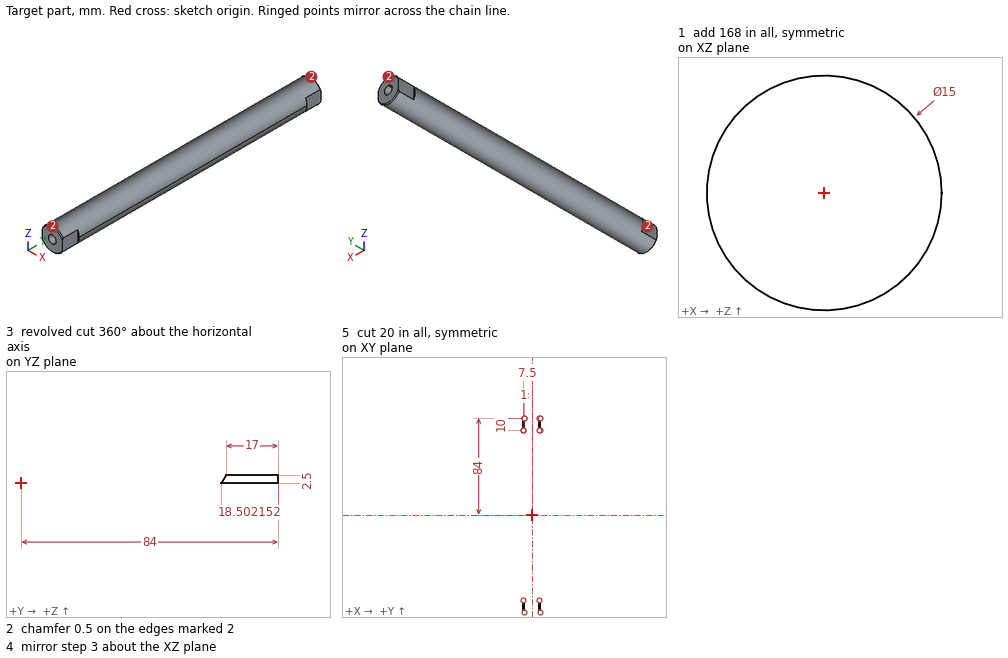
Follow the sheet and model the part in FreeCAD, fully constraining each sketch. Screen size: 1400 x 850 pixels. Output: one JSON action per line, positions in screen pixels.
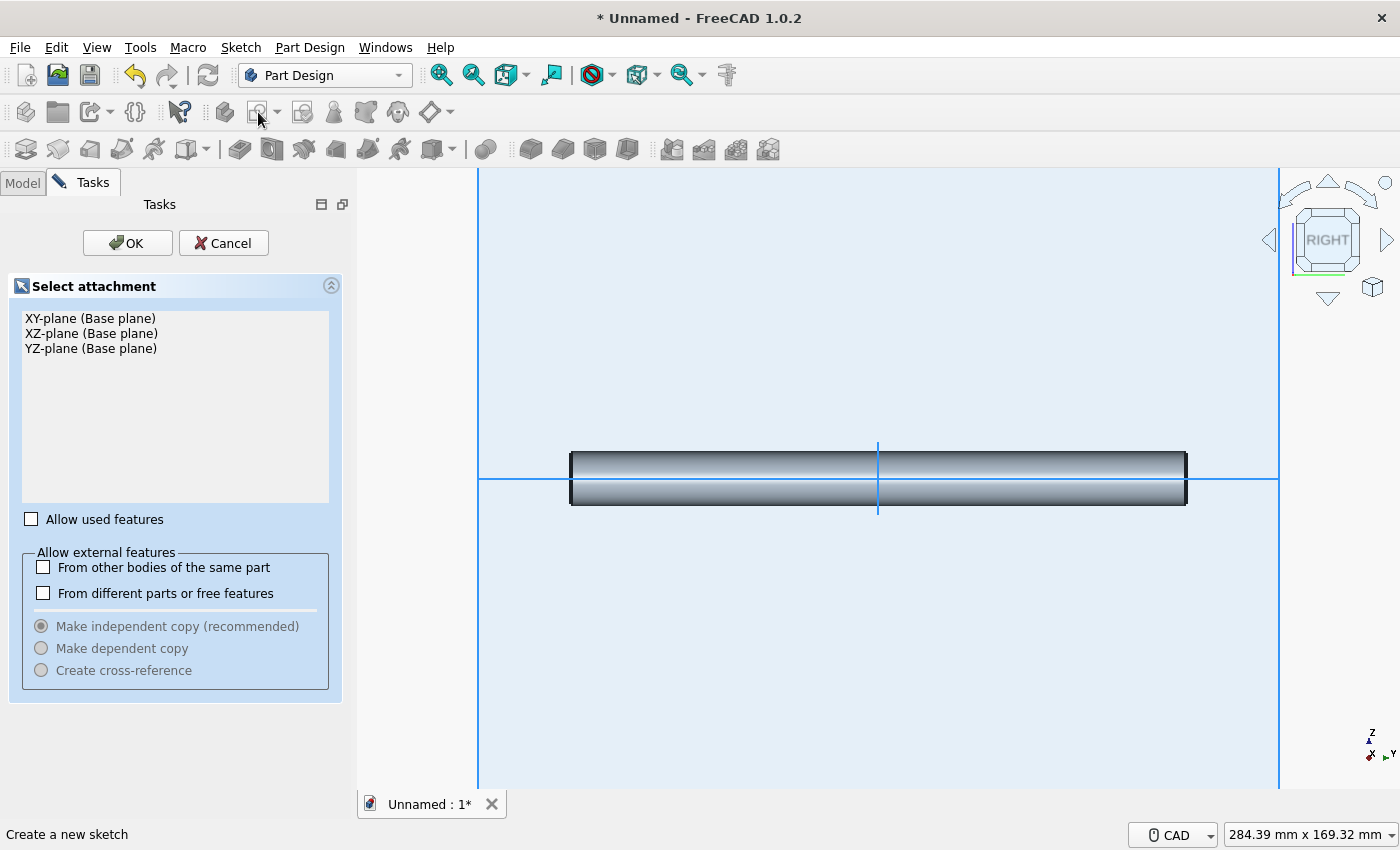
{"action": "left_click", "coordinate": [82, 348]}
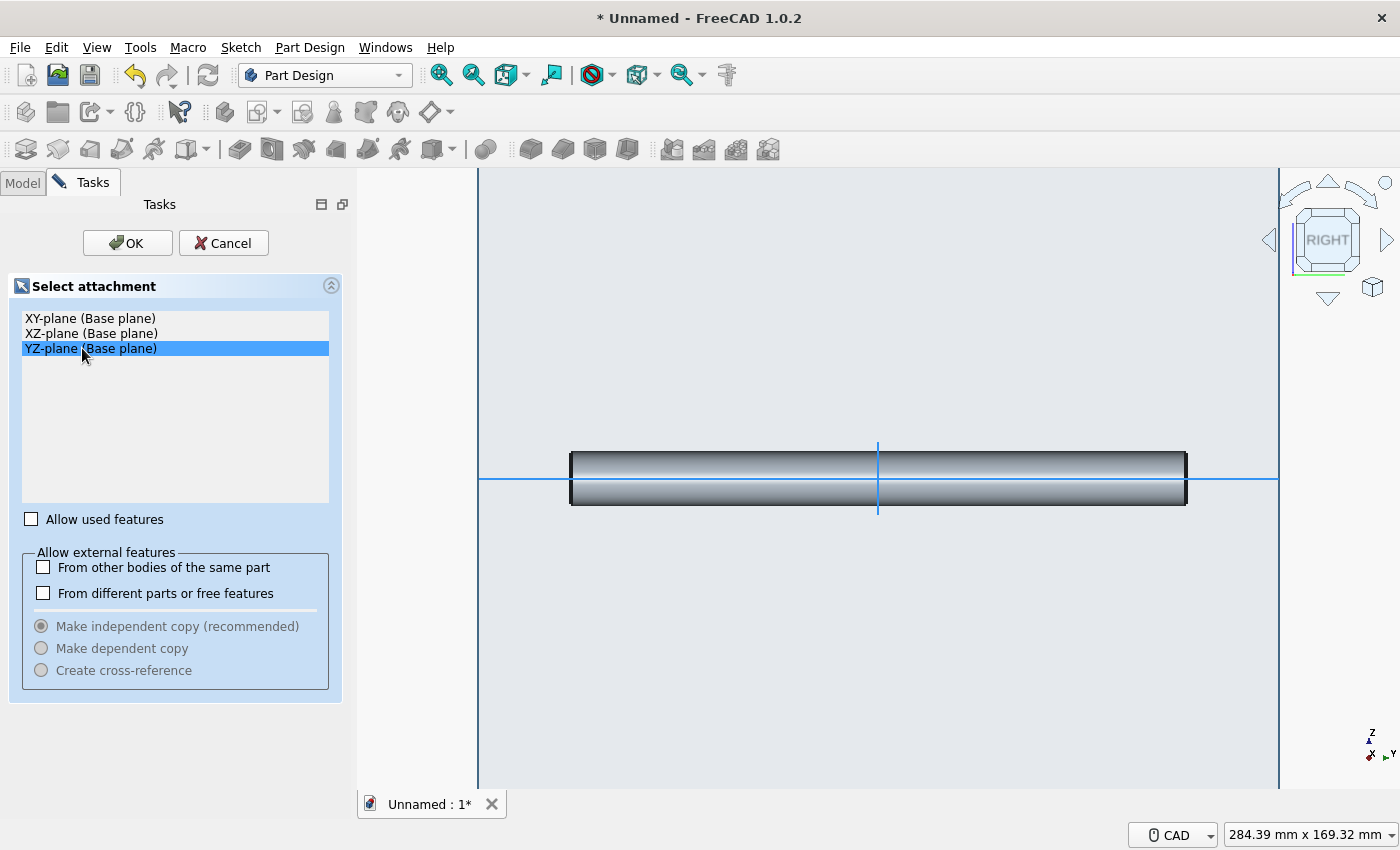
{"action": "left_click", "coordinate": [128, 243]}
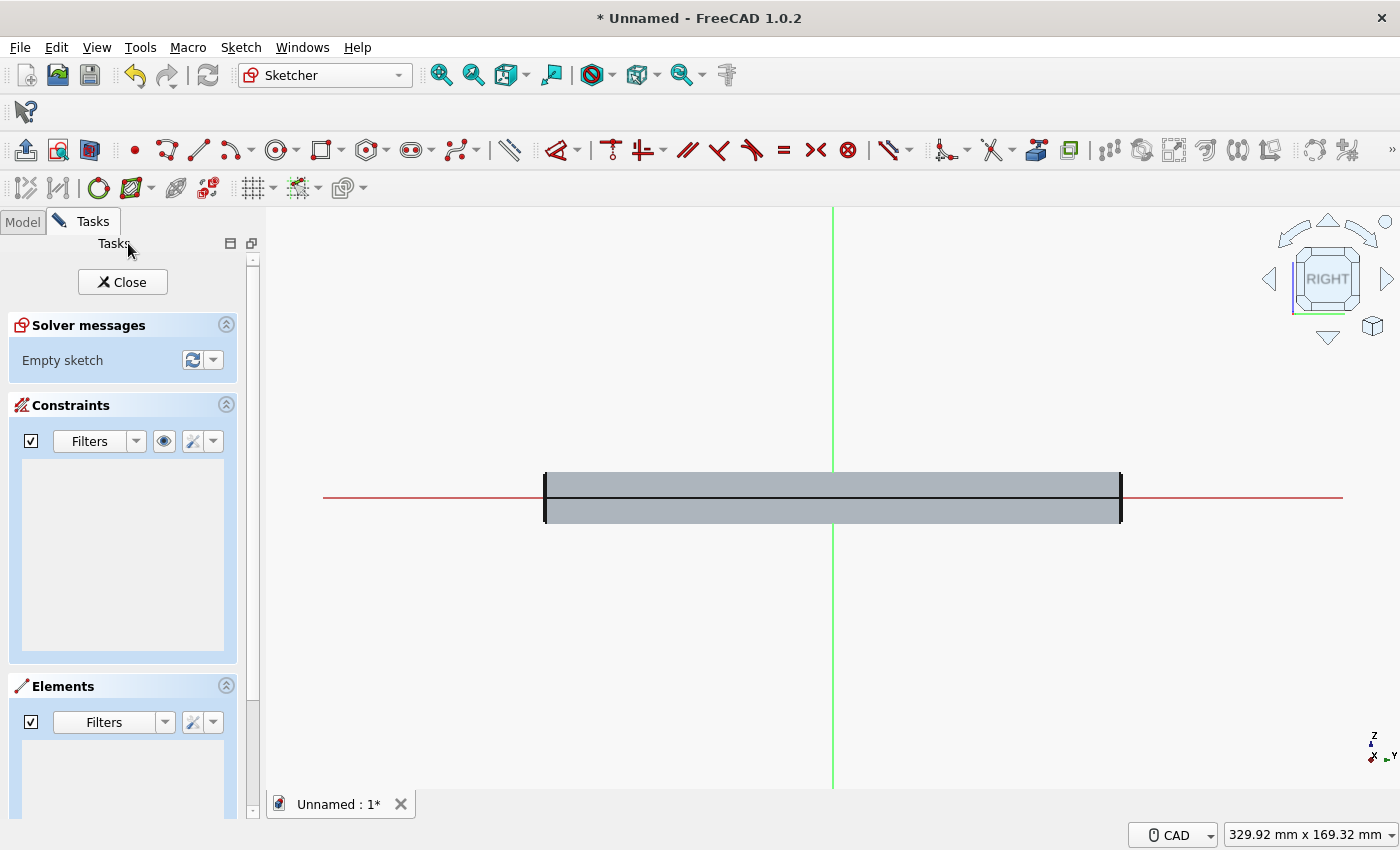
{"action": "left_click", "coordinate": [90, 150]}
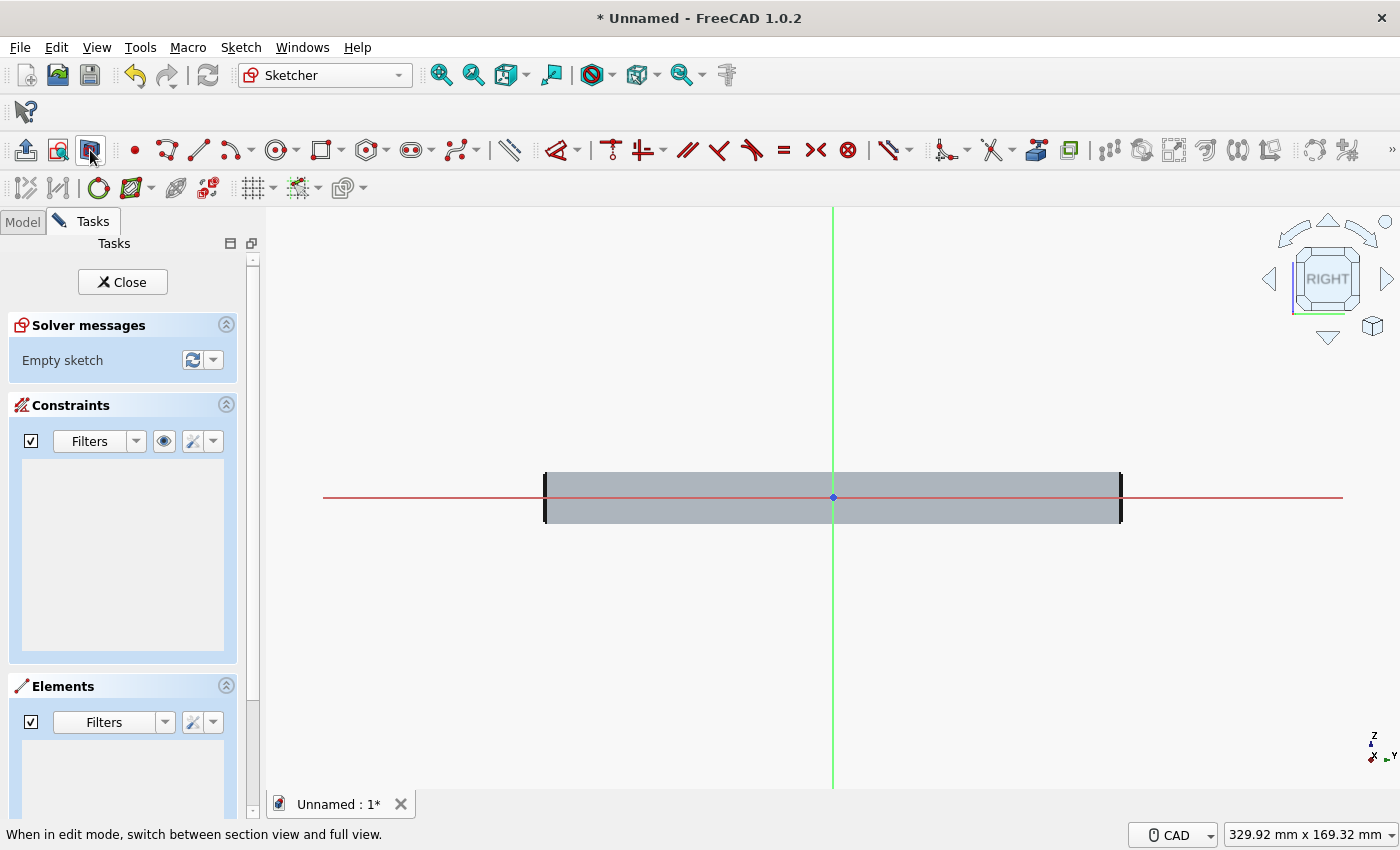
{"action": "scroll", "coordinate": [1122, 493], "scroll_direction": "up", "scroll_amount": 12}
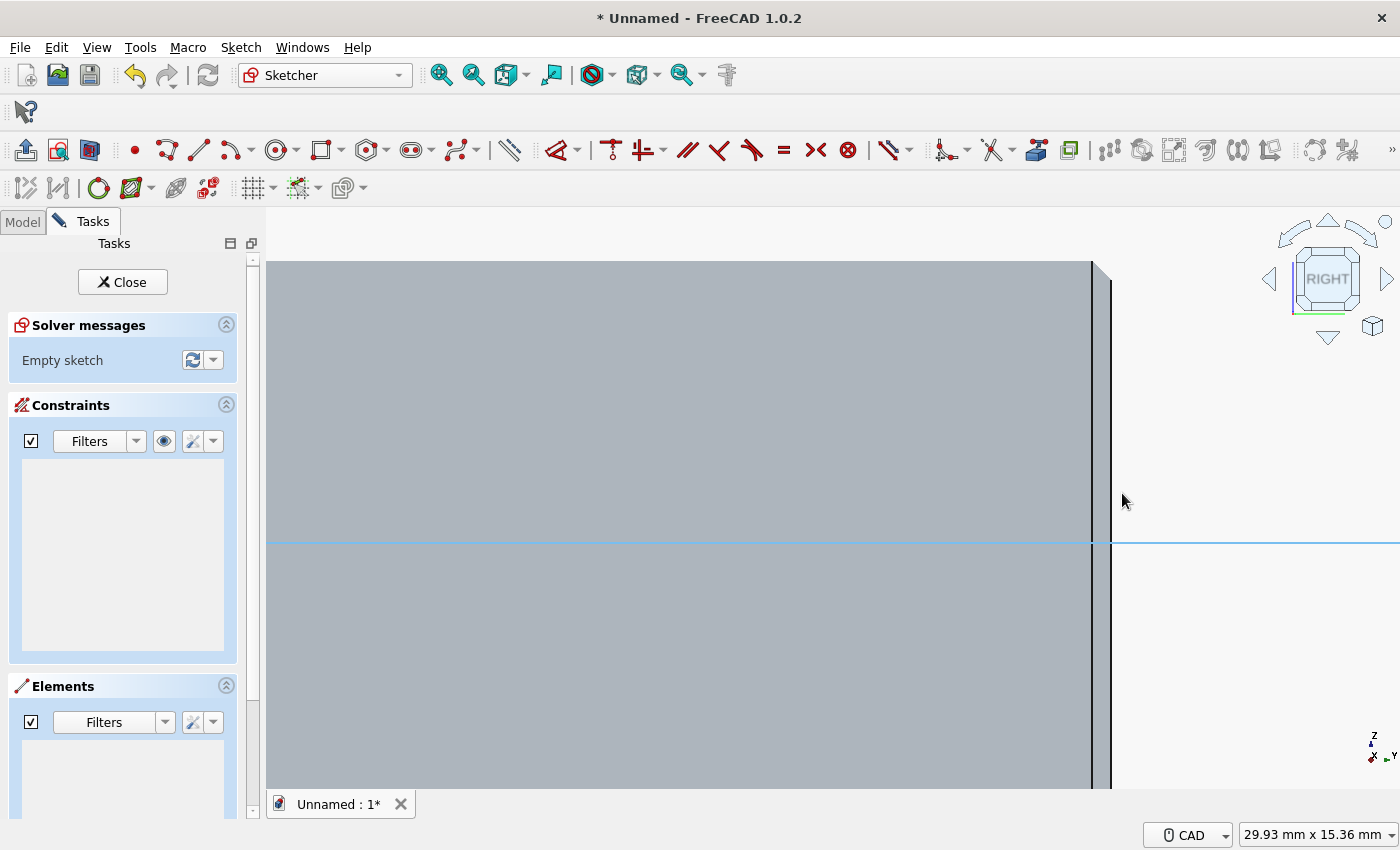
{"action": "left_click", "coordinate": [168, 150]}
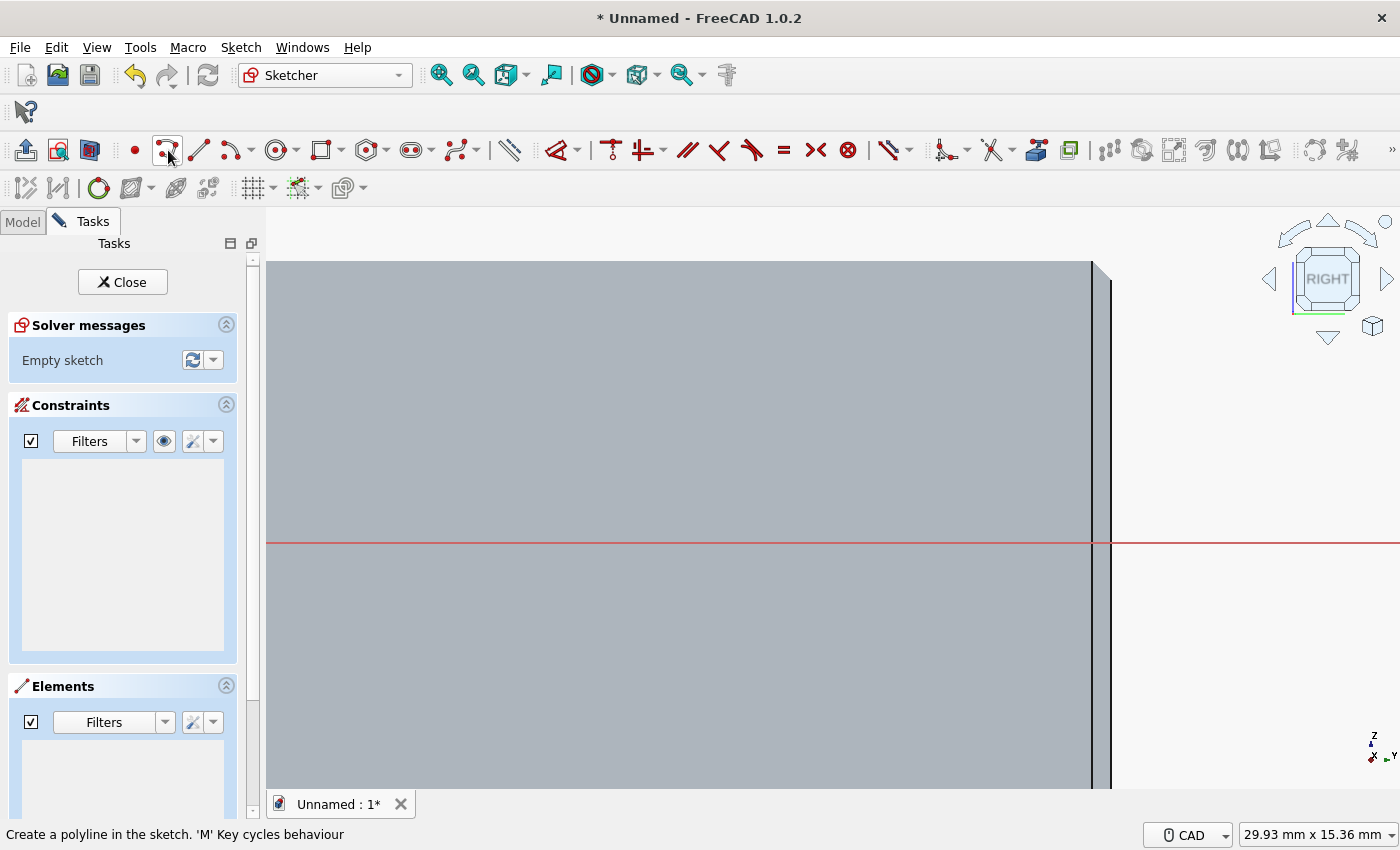
{"action": "left_click", "coordinate": [410, 543]}
{"action": "left_click", "coordinate": [1111, 534]}
{"action": "left_click", "coordinate": [1111, 448]}
{"action": "left_click", "coordinate": [467, 448]}
{"action": "left_click", "coordinate": [410, 543]}
{"action": "key", "text": "Escape"}
{"action": "key", "text": "Escape"}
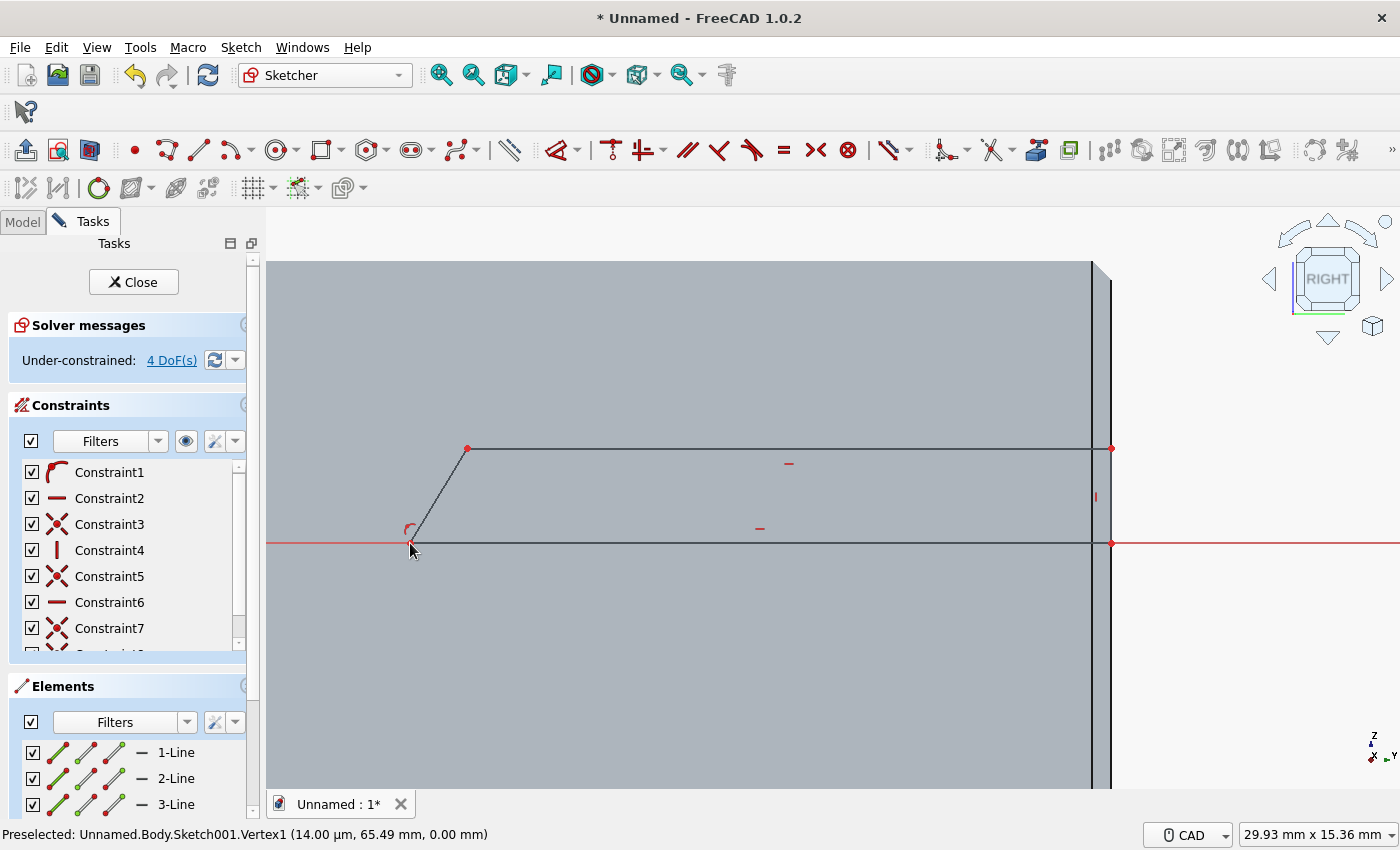
{"action": "left_click", "coordinate": [556, 150]}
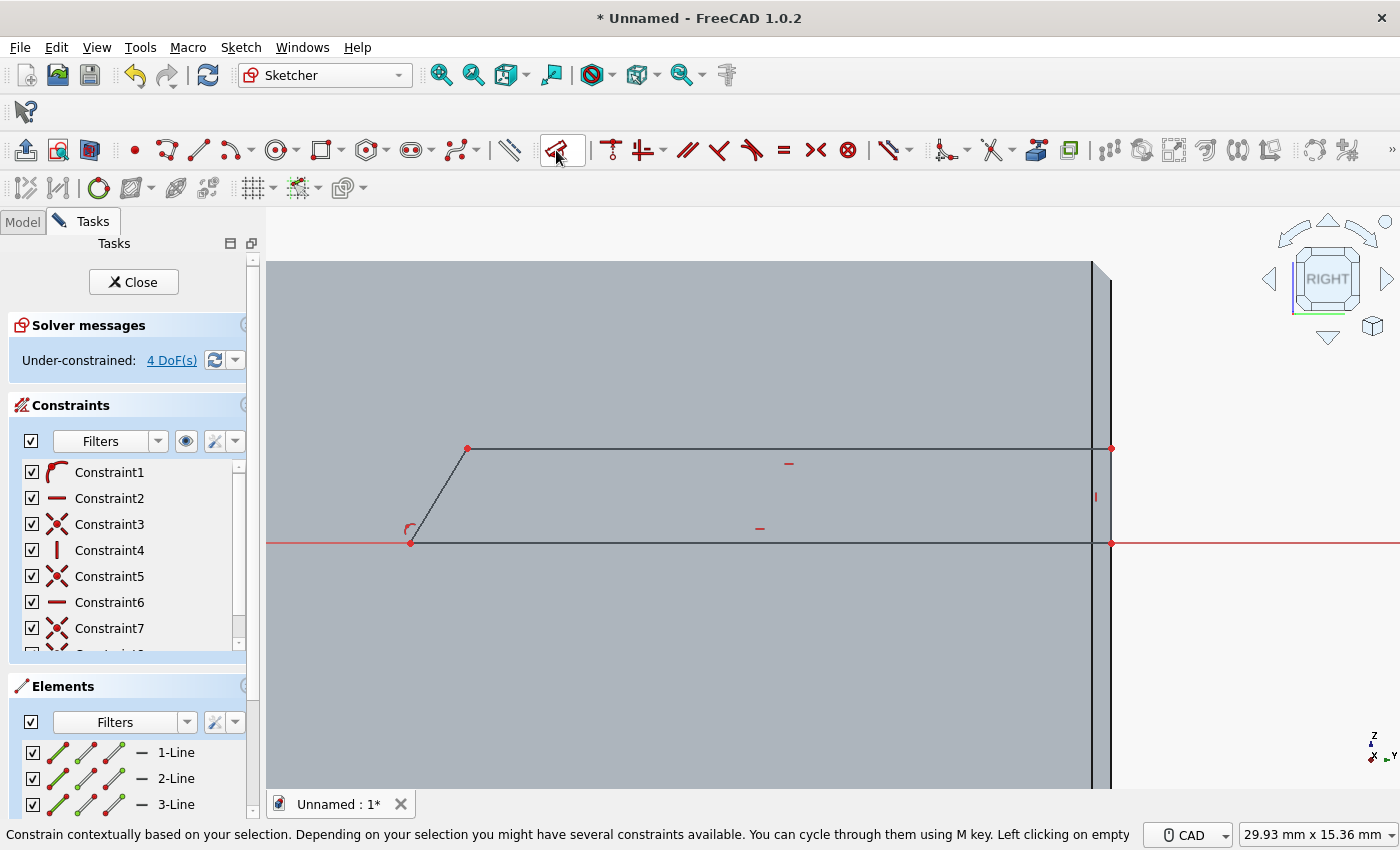
{"action": "left_click", "coordinate": [918, 449]}
{"action": "left_click", "coordinate": [789, 415]}